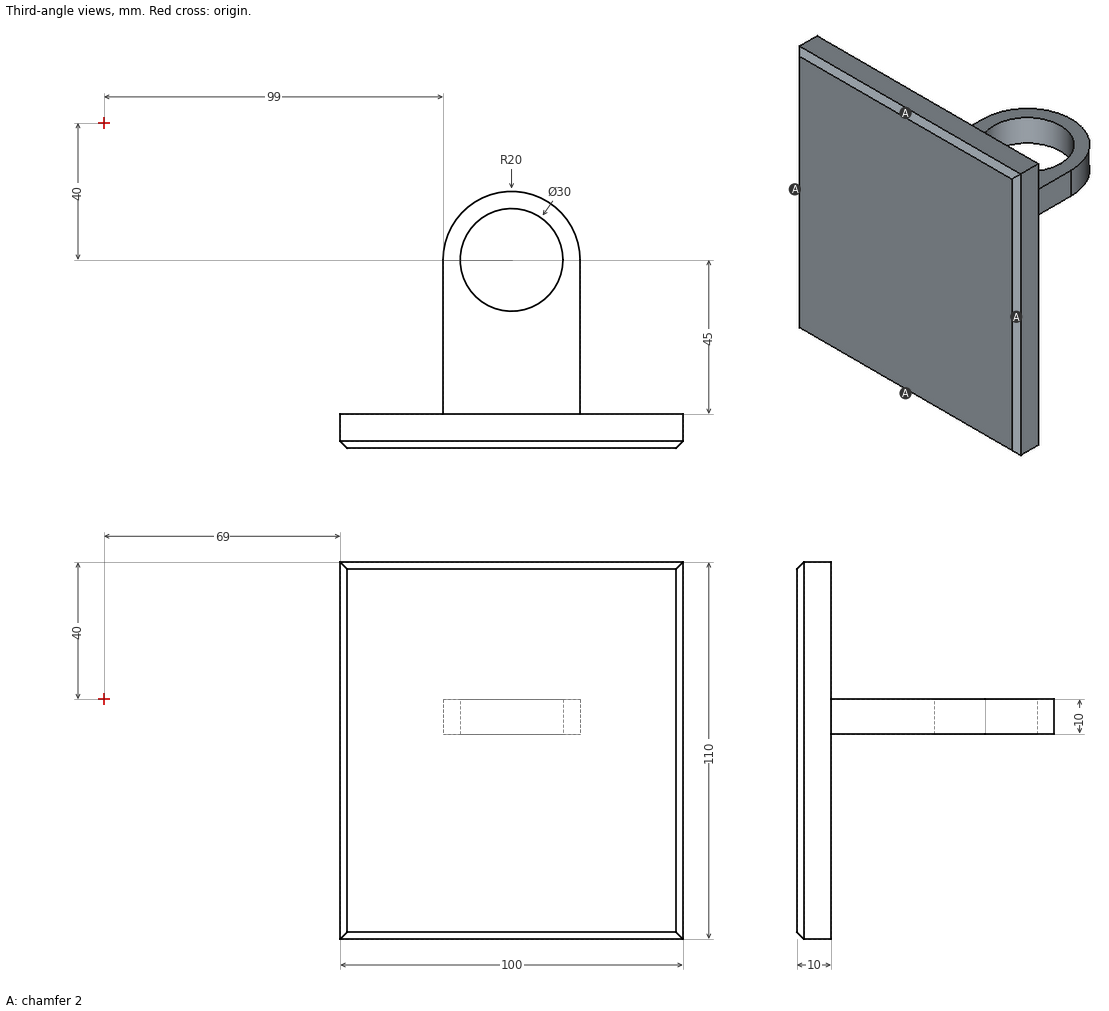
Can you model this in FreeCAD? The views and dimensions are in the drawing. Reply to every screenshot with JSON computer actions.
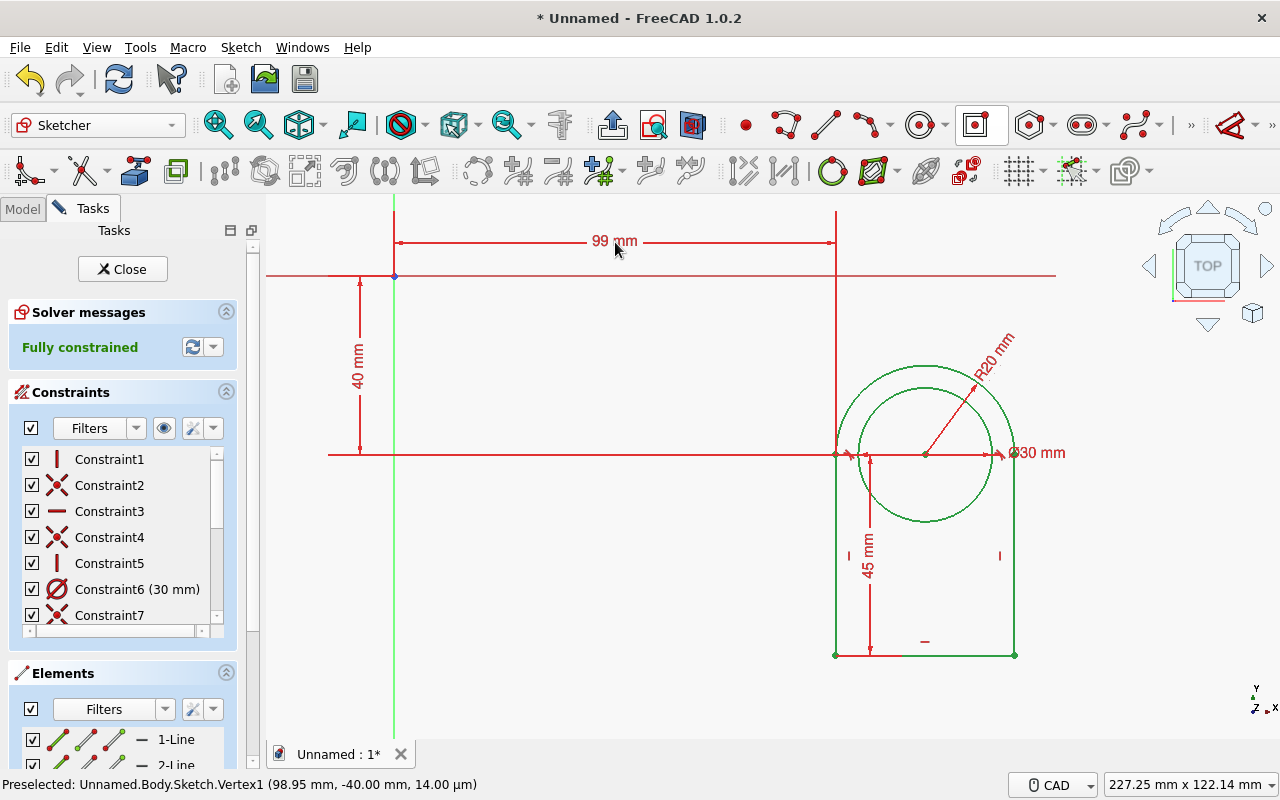
{"action": "left_click", "coordinate": [123, 269]}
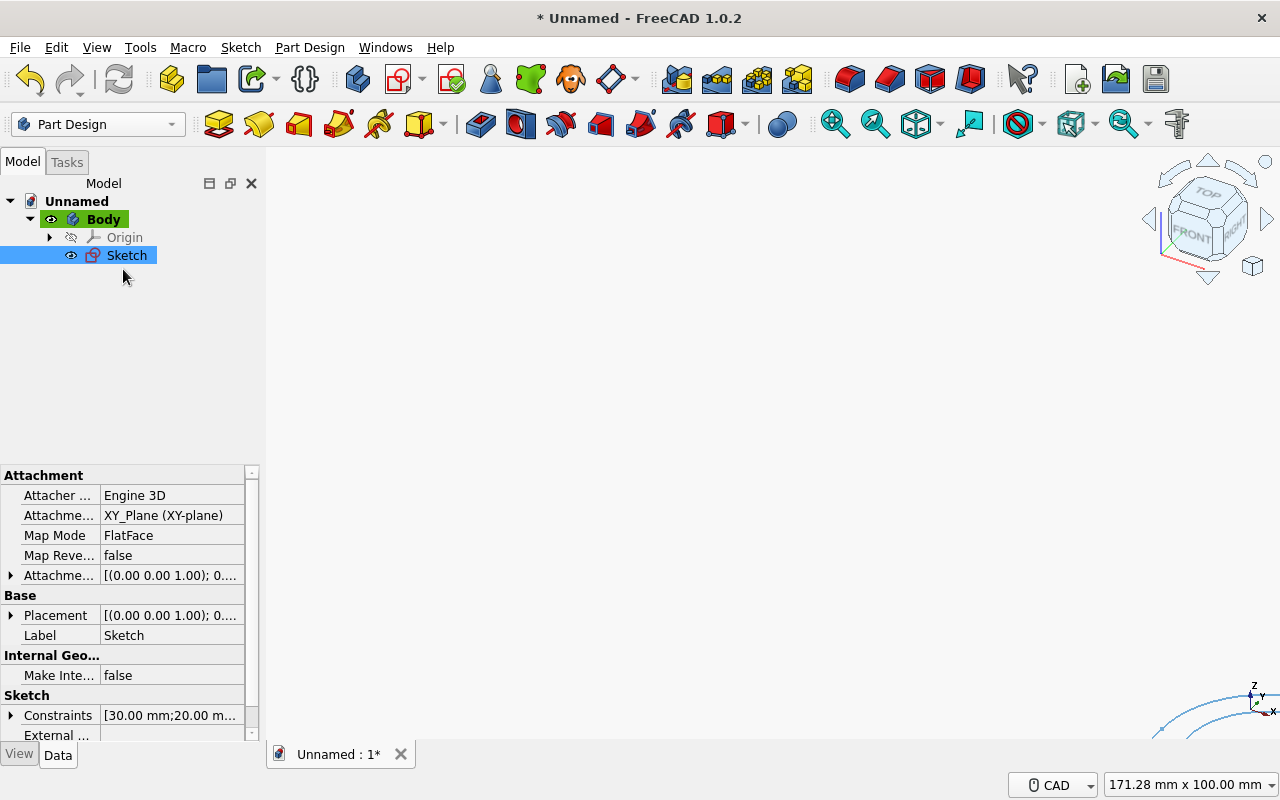
{"action": "left_click", "coordinate": [220, 124]}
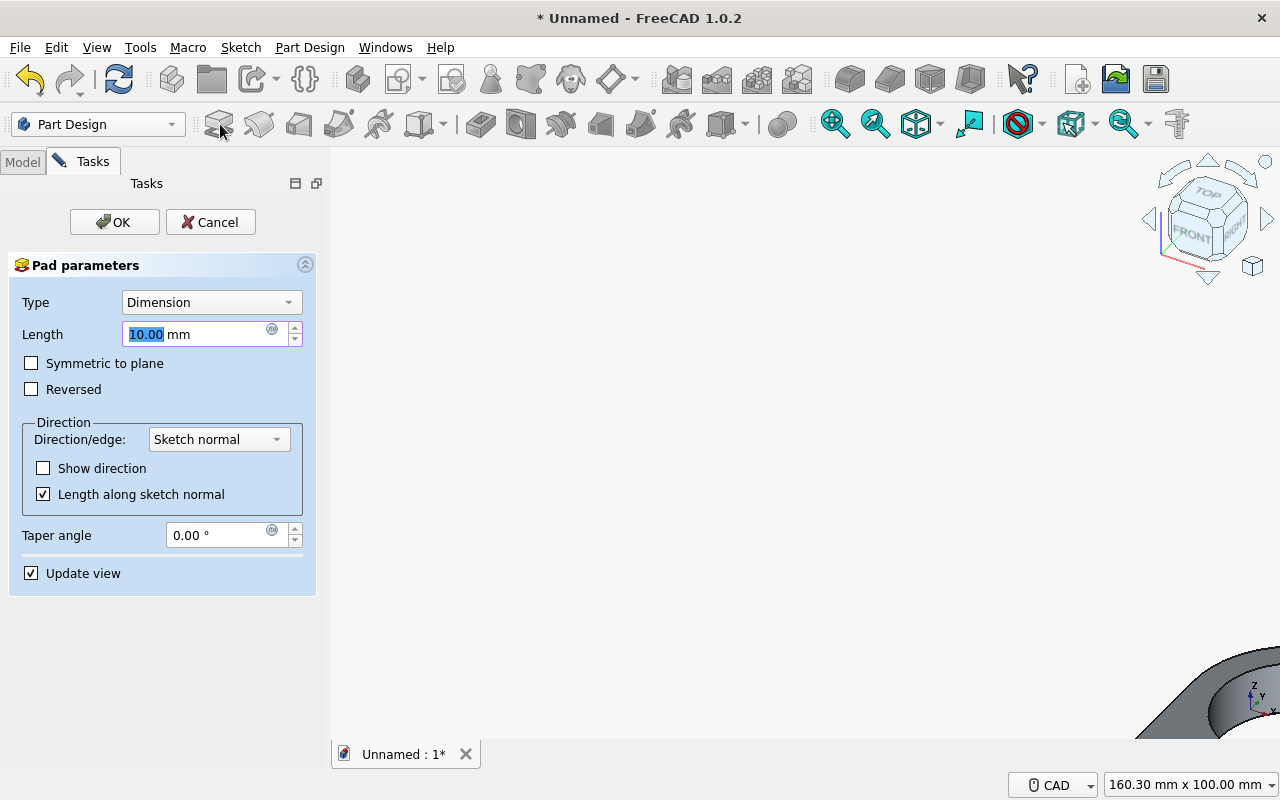
{"action": "type", "text": "10"}
{"action": "key", "text": "Tab"}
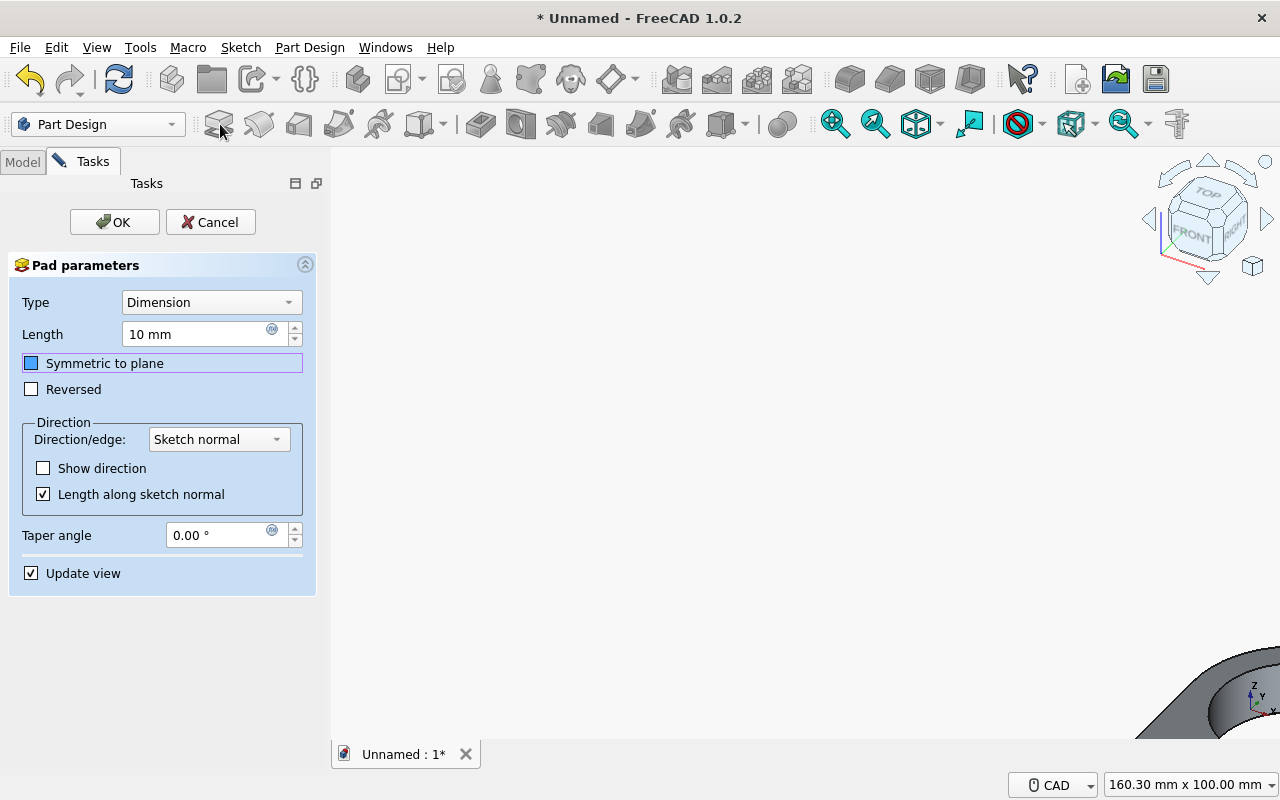
{"action": "left_click", "coordinate": [30, 389]}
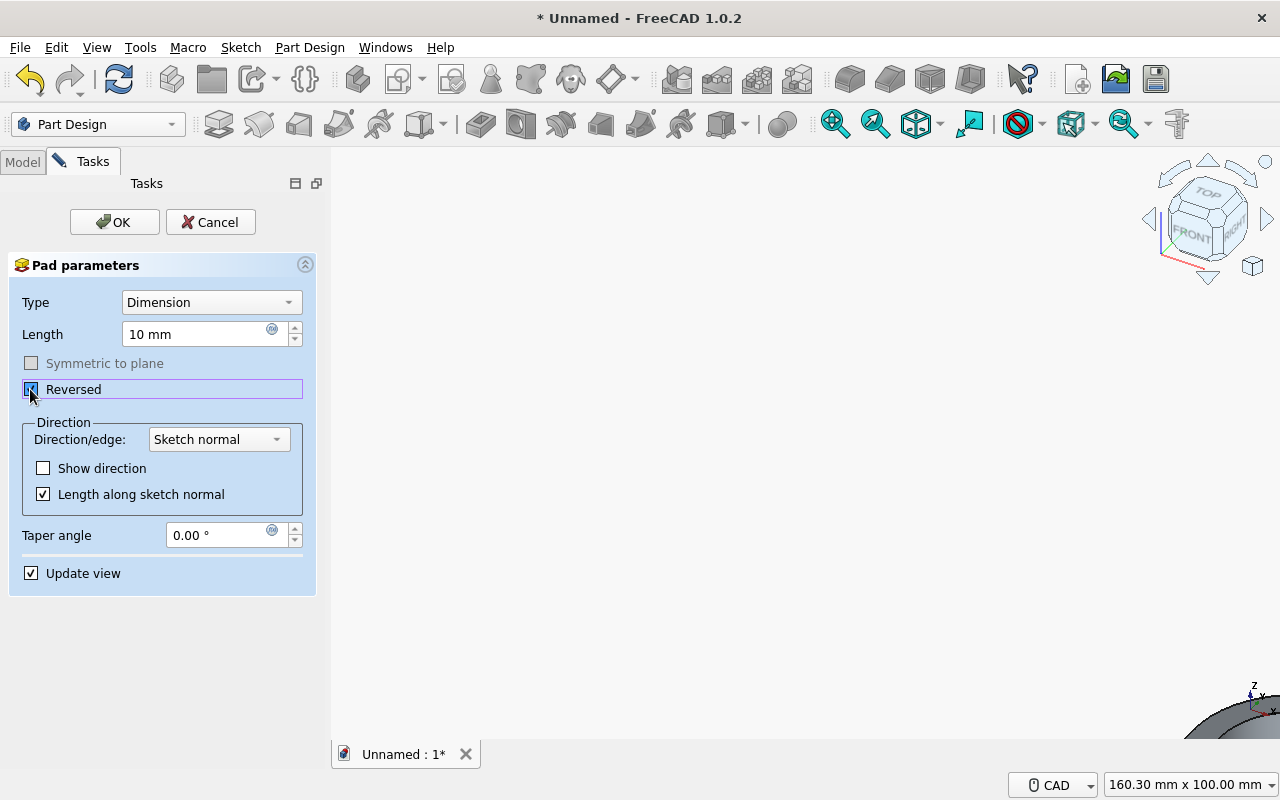
{"action": "left_click", "coordinate": [115, 222]}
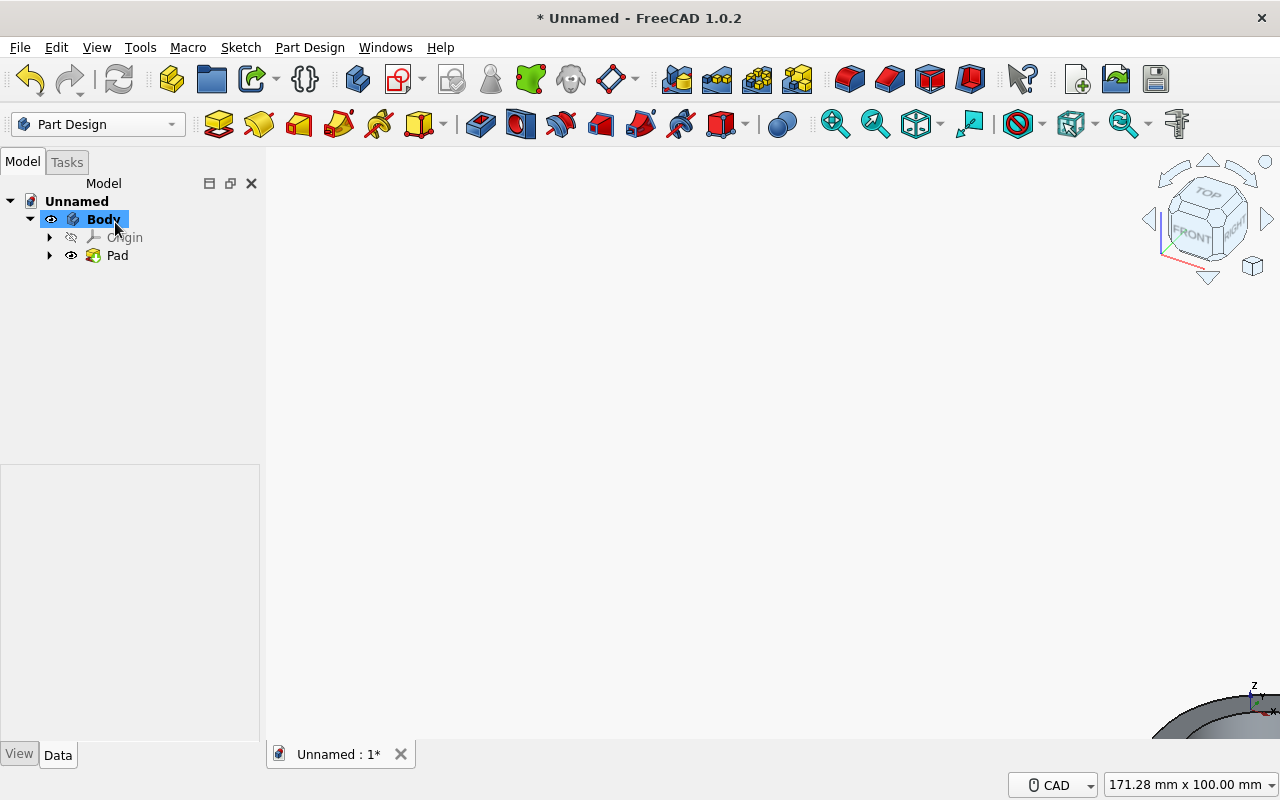
{"action": "left_click", "coordinate": [836, 124]}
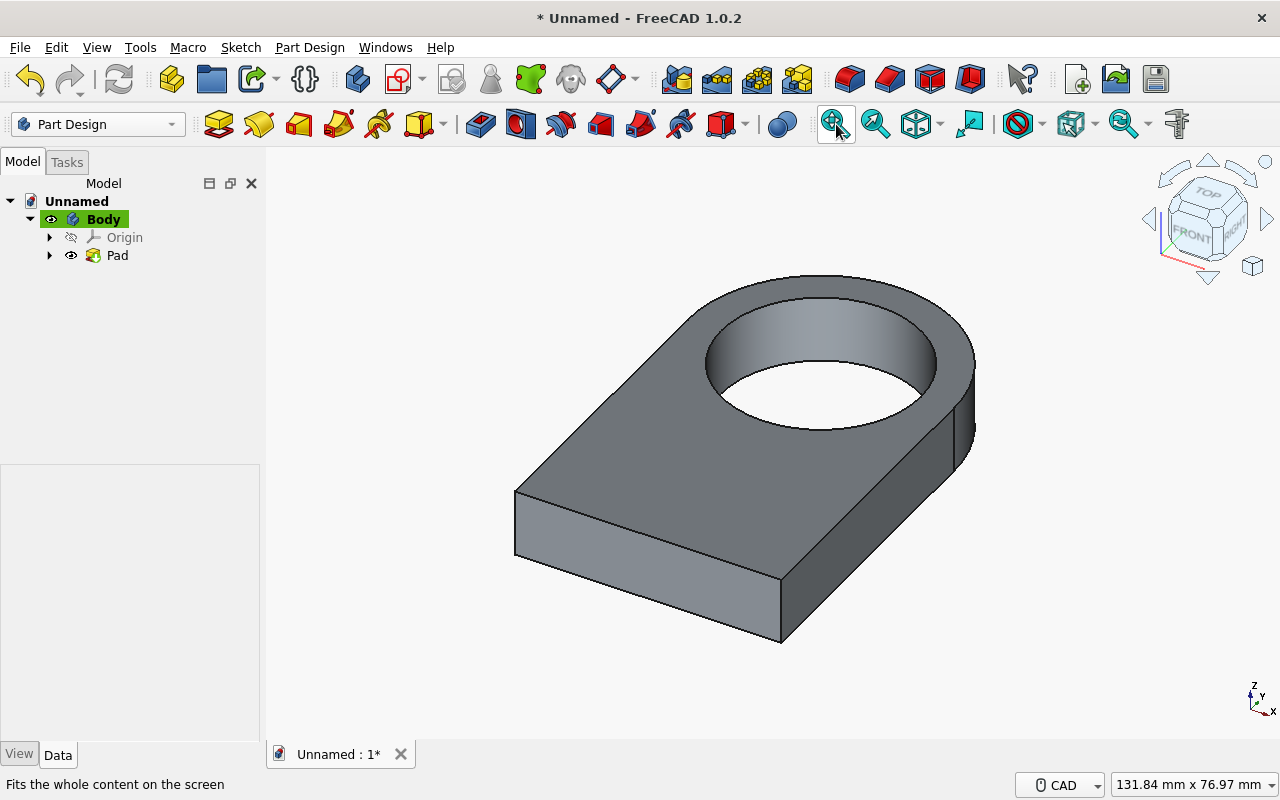
{"action": "left_click", "coordinate": [724, 591]}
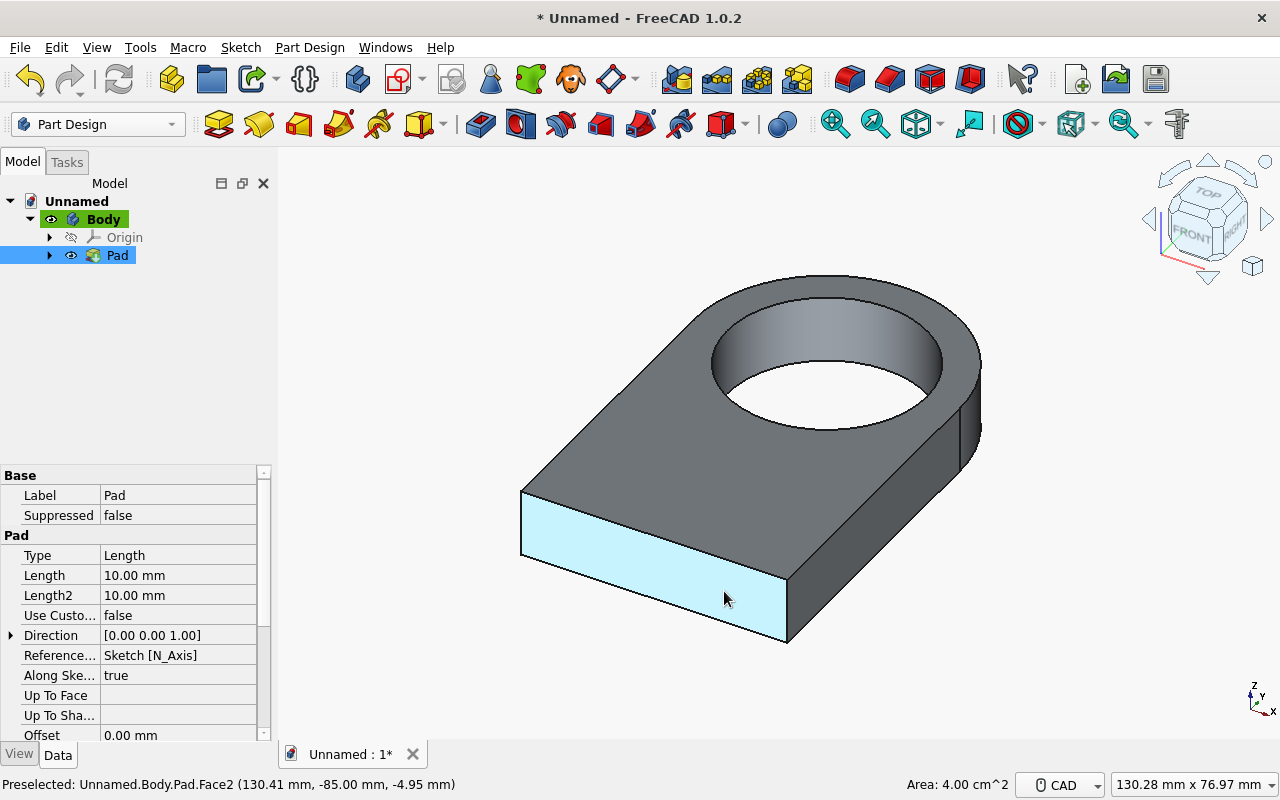
{"action": "left_click", "coordinate": [398, 80]}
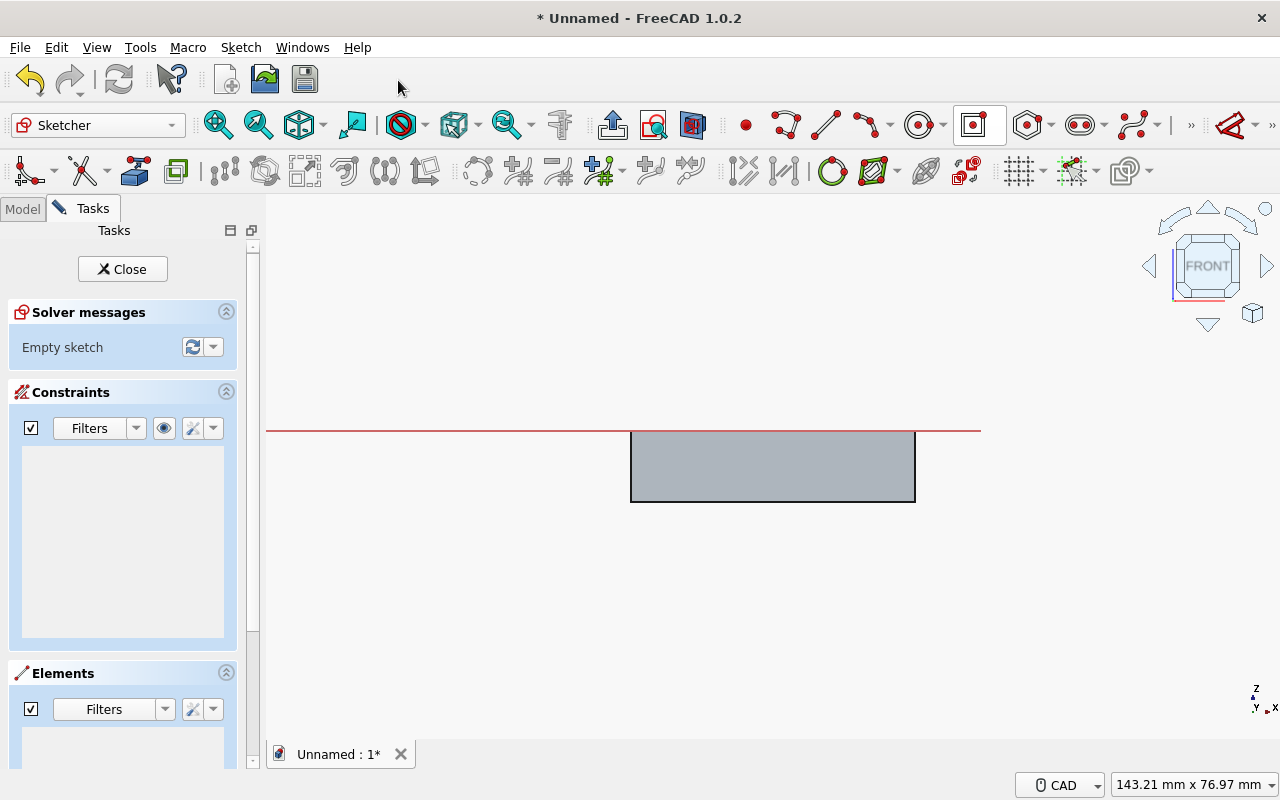
{"action": "scroll", "coordinate": [848, 409], "scroll_direction": "down", "scroll_amount": 4}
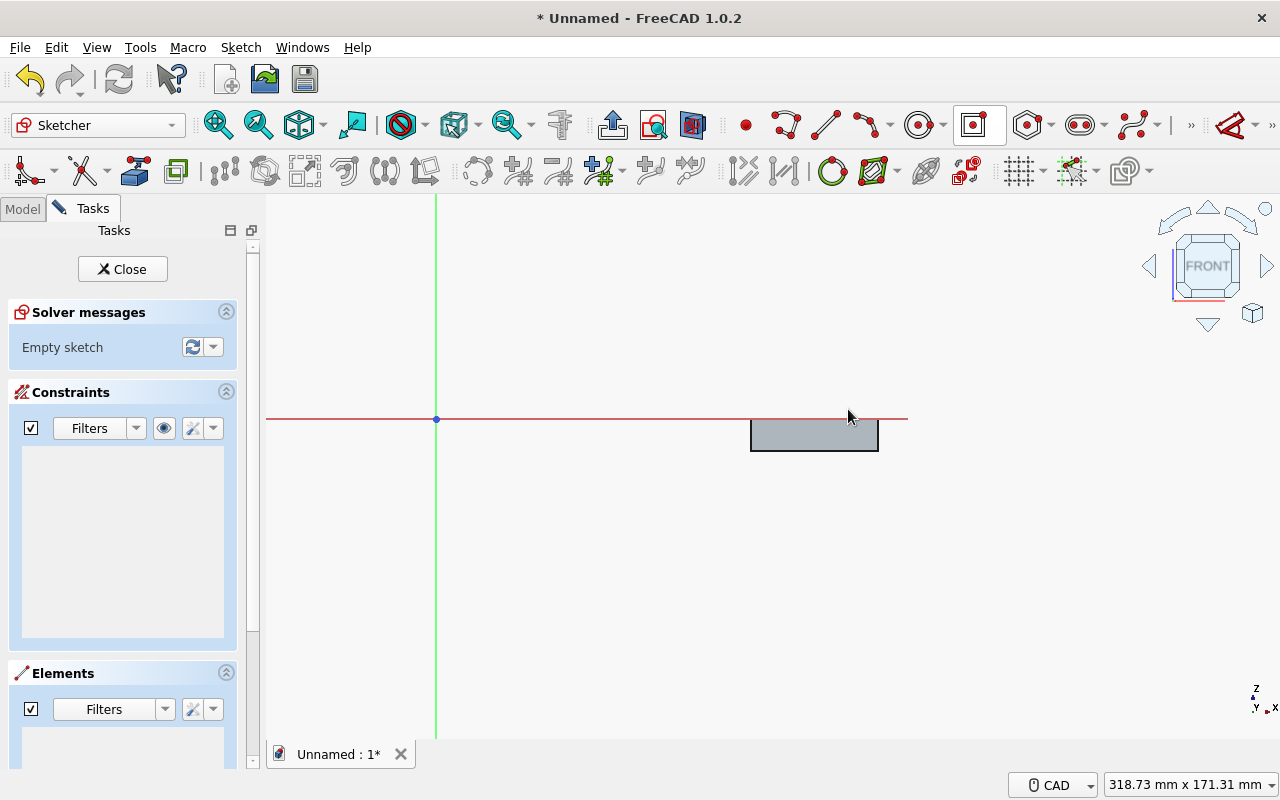
{"action": "left_click", "coordinate": [1000, 126]}